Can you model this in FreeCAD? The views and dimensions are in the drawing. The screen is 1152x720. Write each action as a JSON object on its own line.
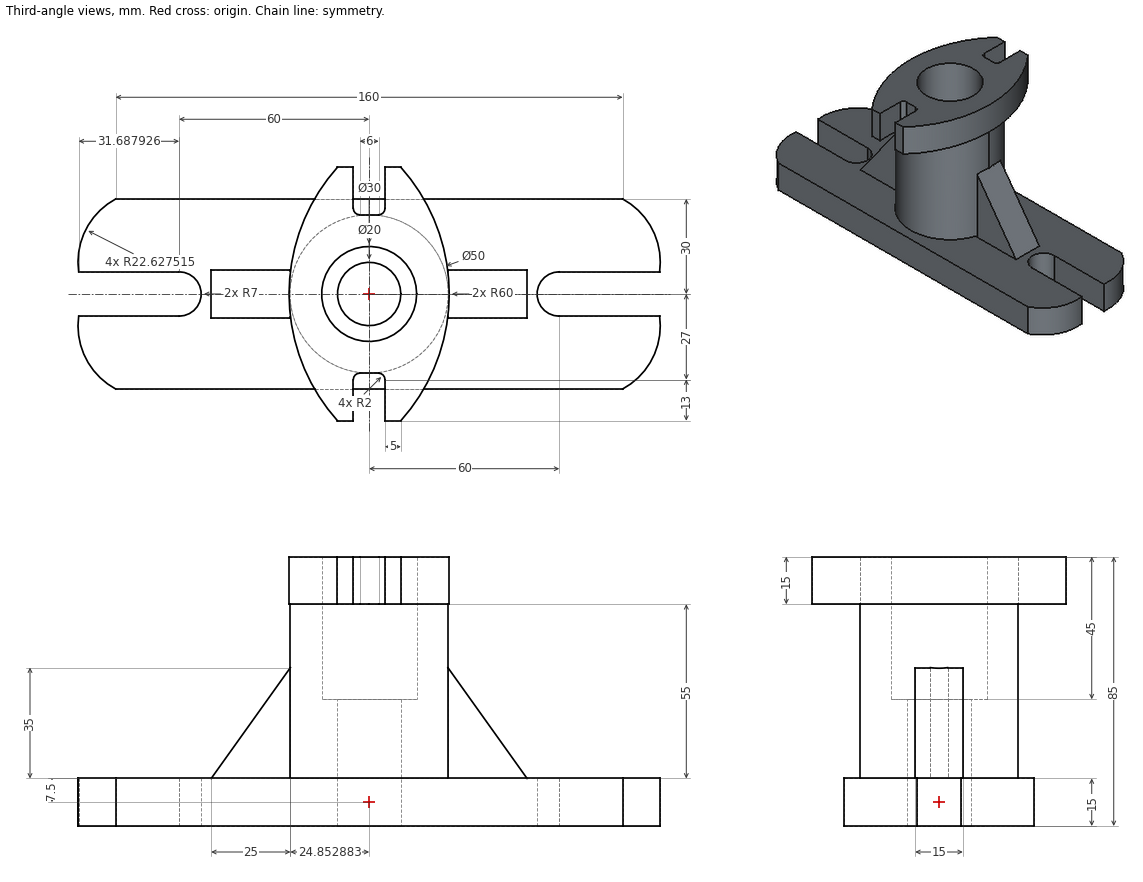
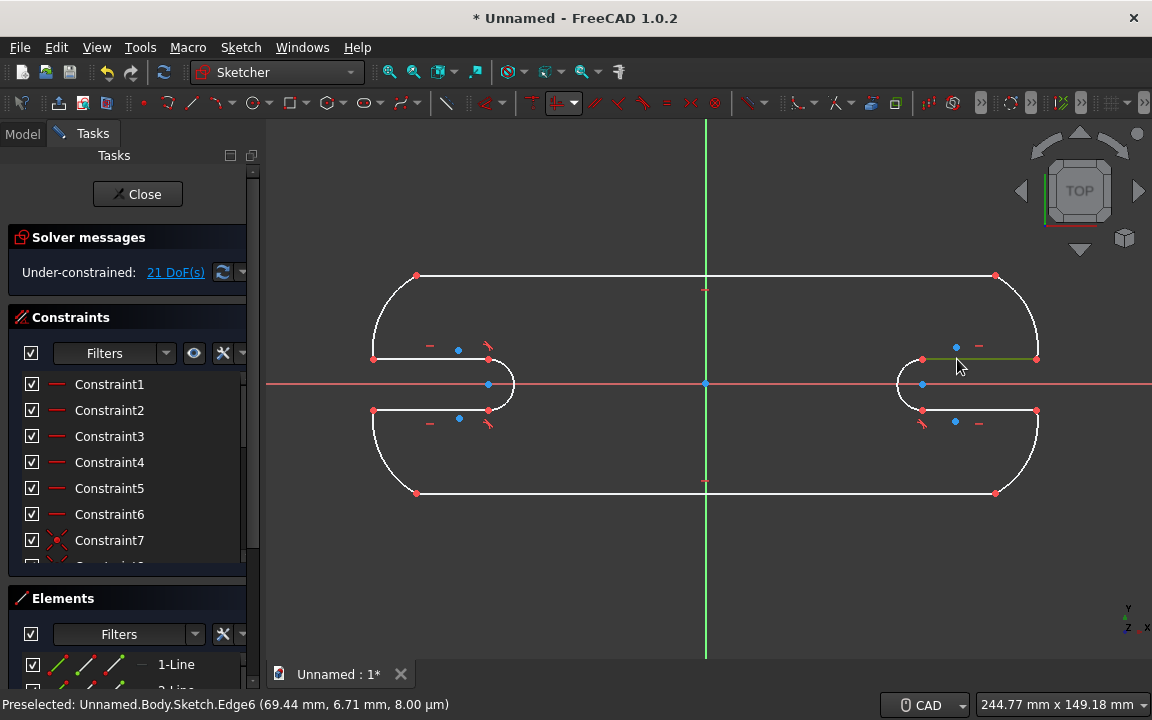
{"action": "left_click", "coordinate": [902, 370]}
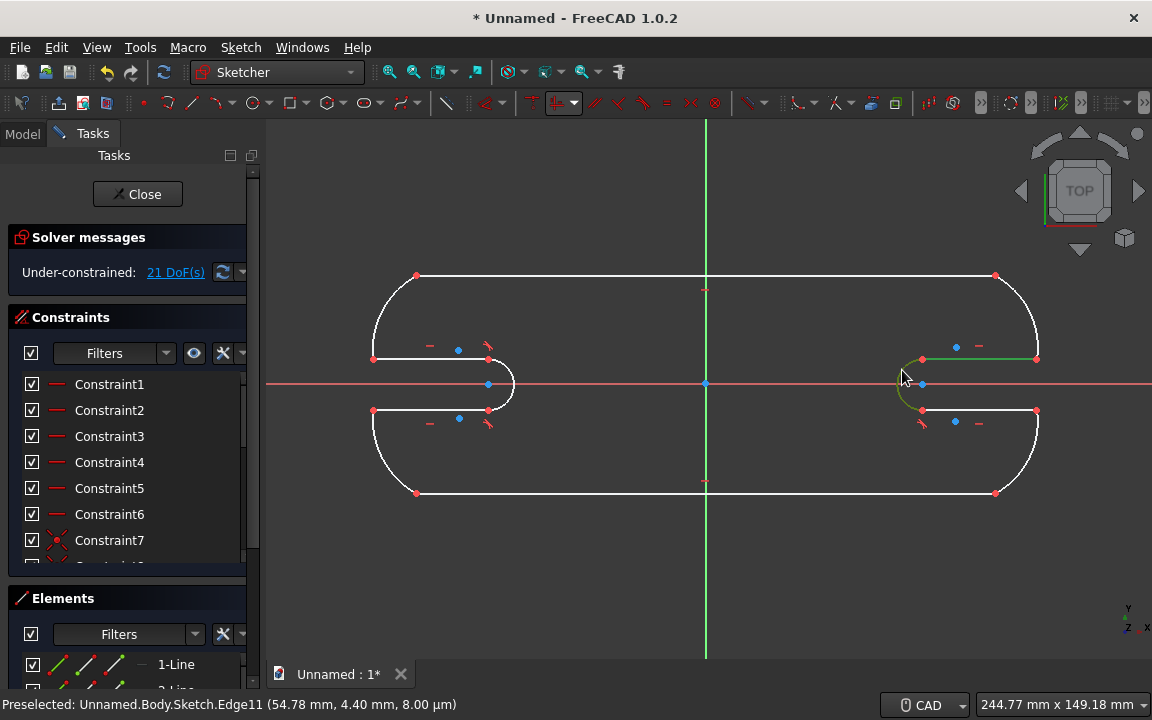
{"action": "key", "text": "t"}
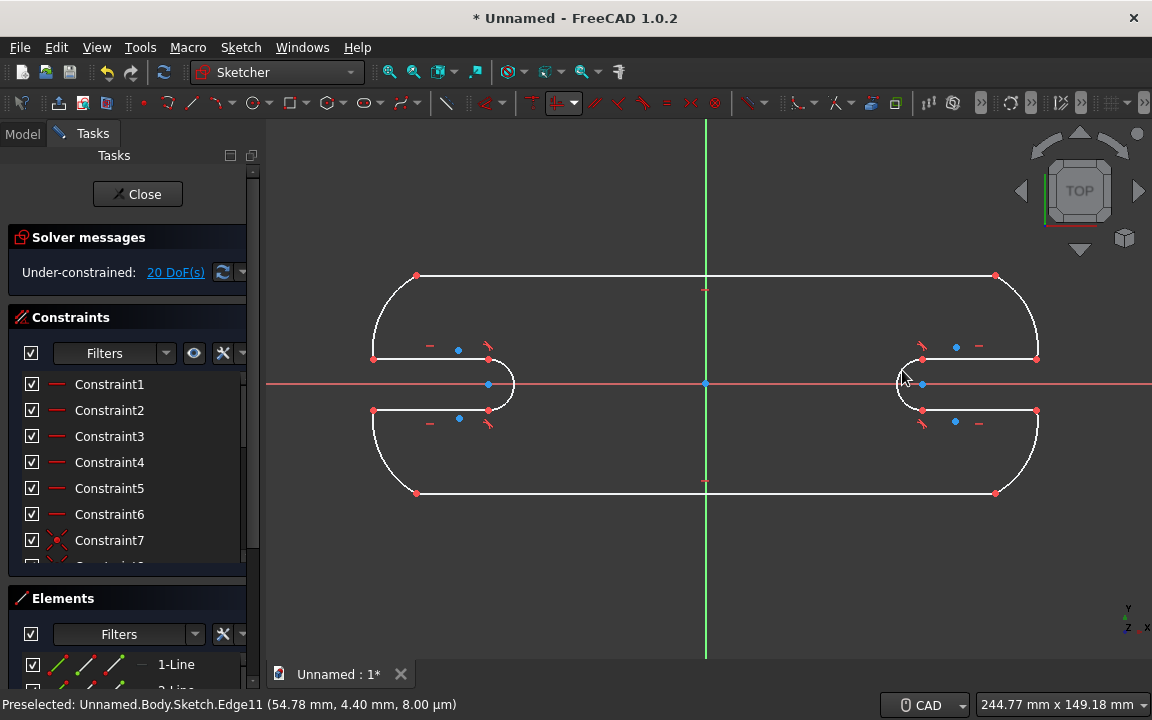
{"action": "left_click", "coordinate": [393, 295]}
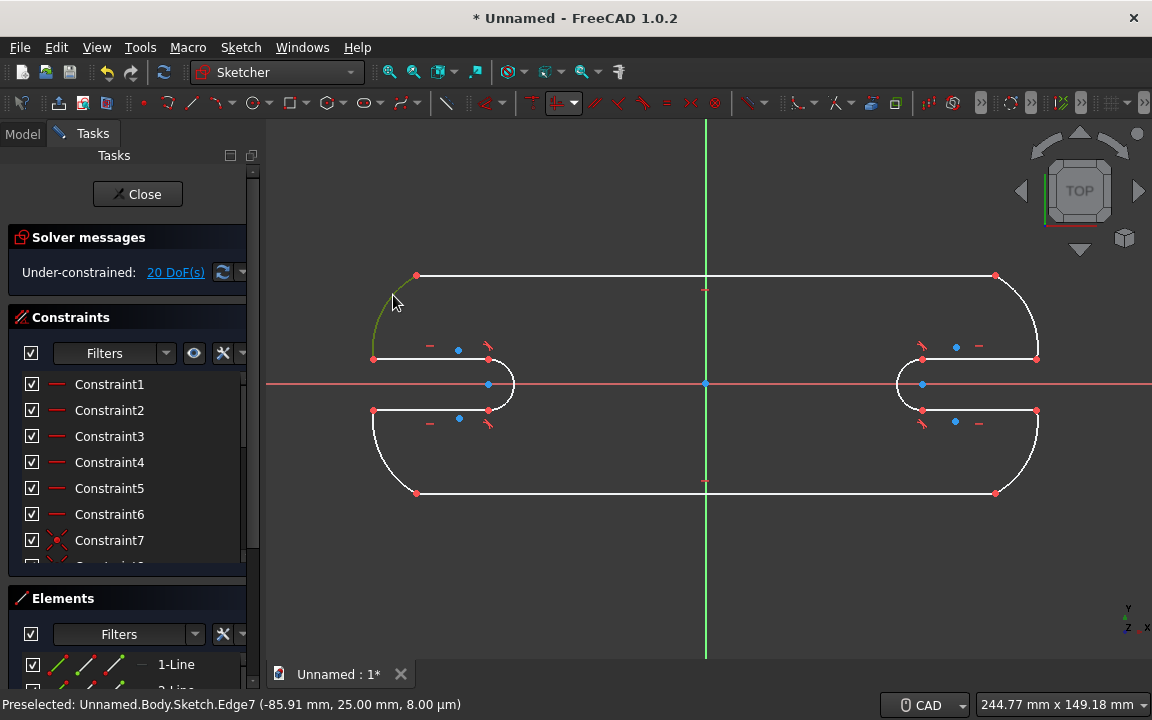
{"action": "left_click", "coordinate": [375, 440]}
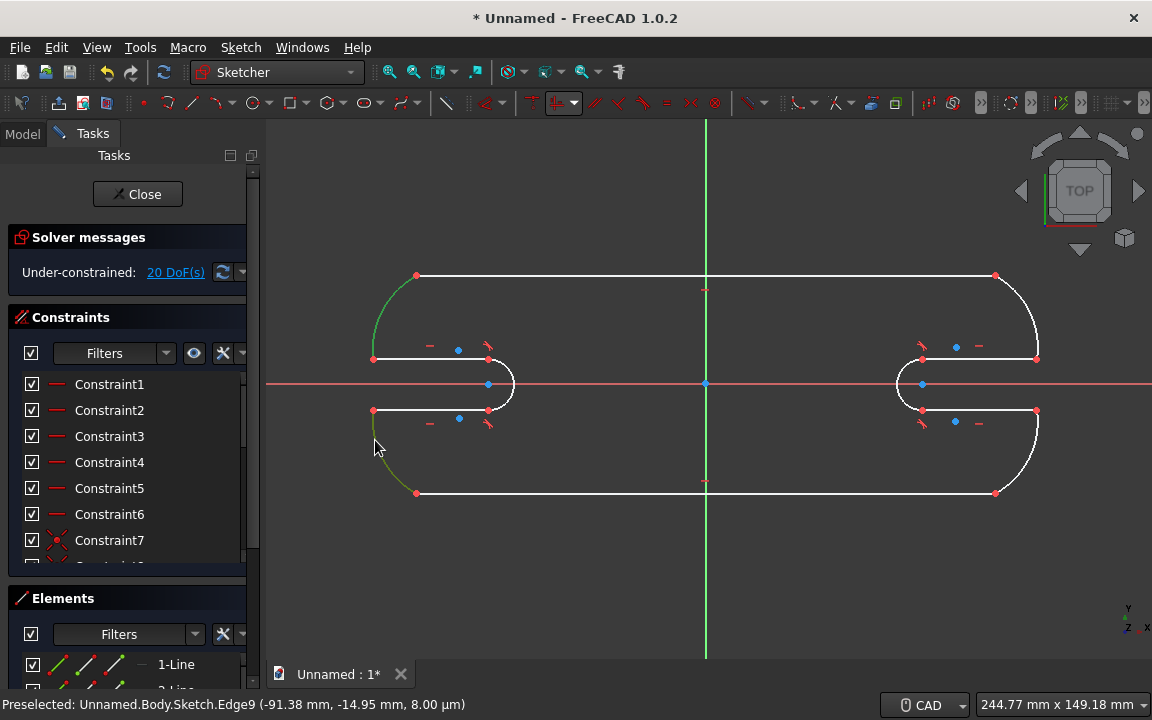
{"action": "scroll", "coordinate": [508, 400], "scroll_direction": "down", "scroll_amount": 2}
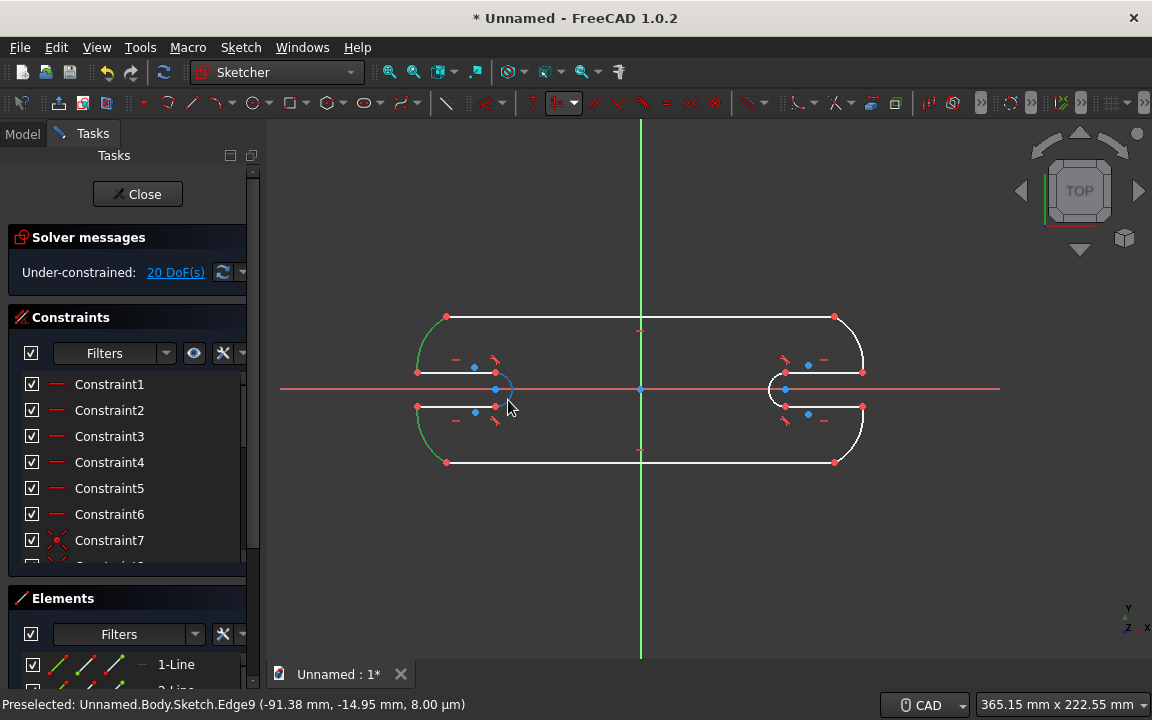
{"action": "left_click", "coordinate": [850, 450]}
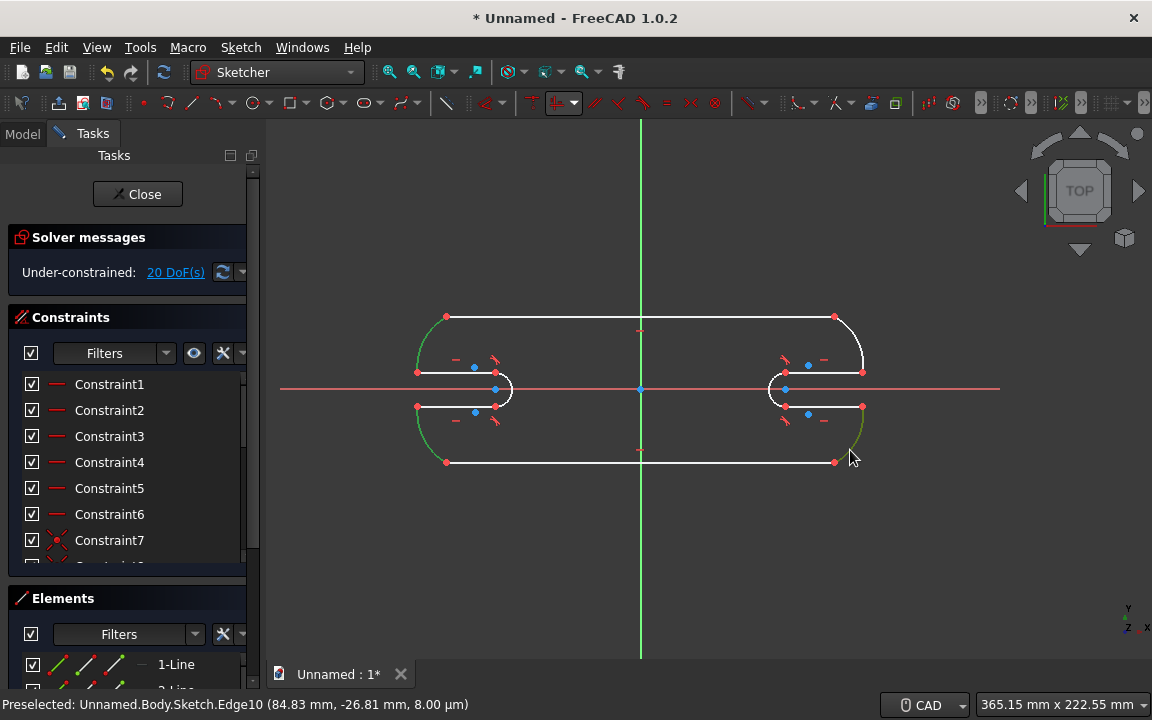
{"action": "left_click", "coordinate": [862, 353]}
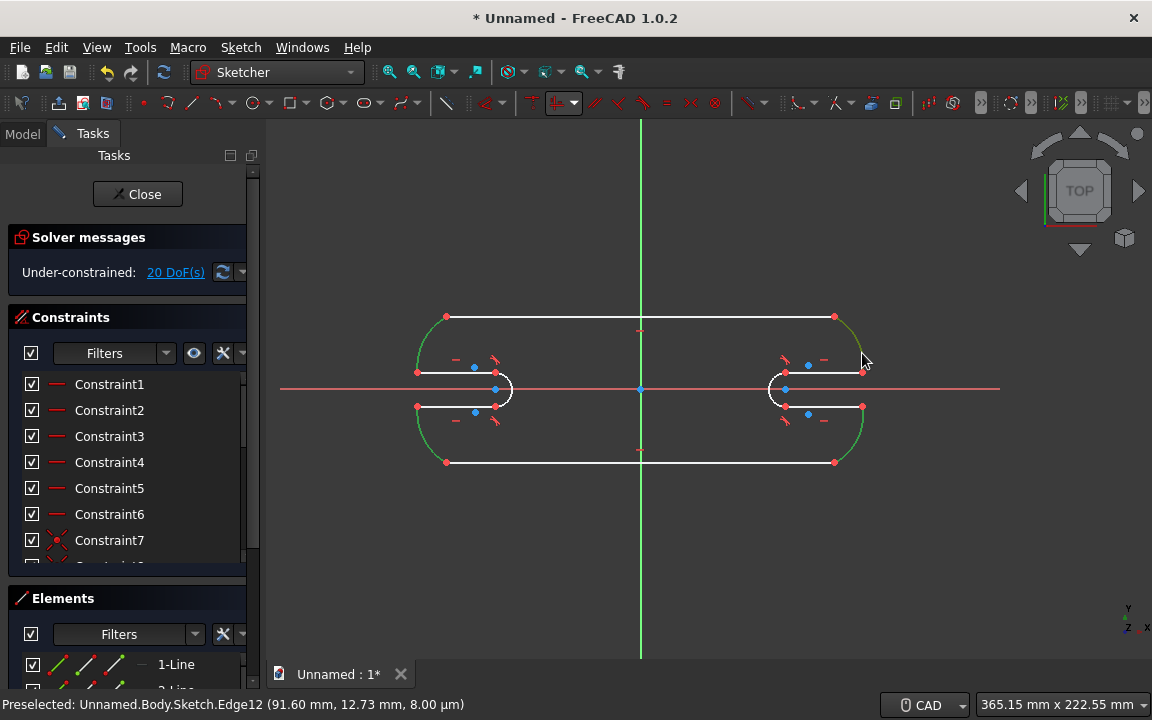
{"action": "key", "text": "e"}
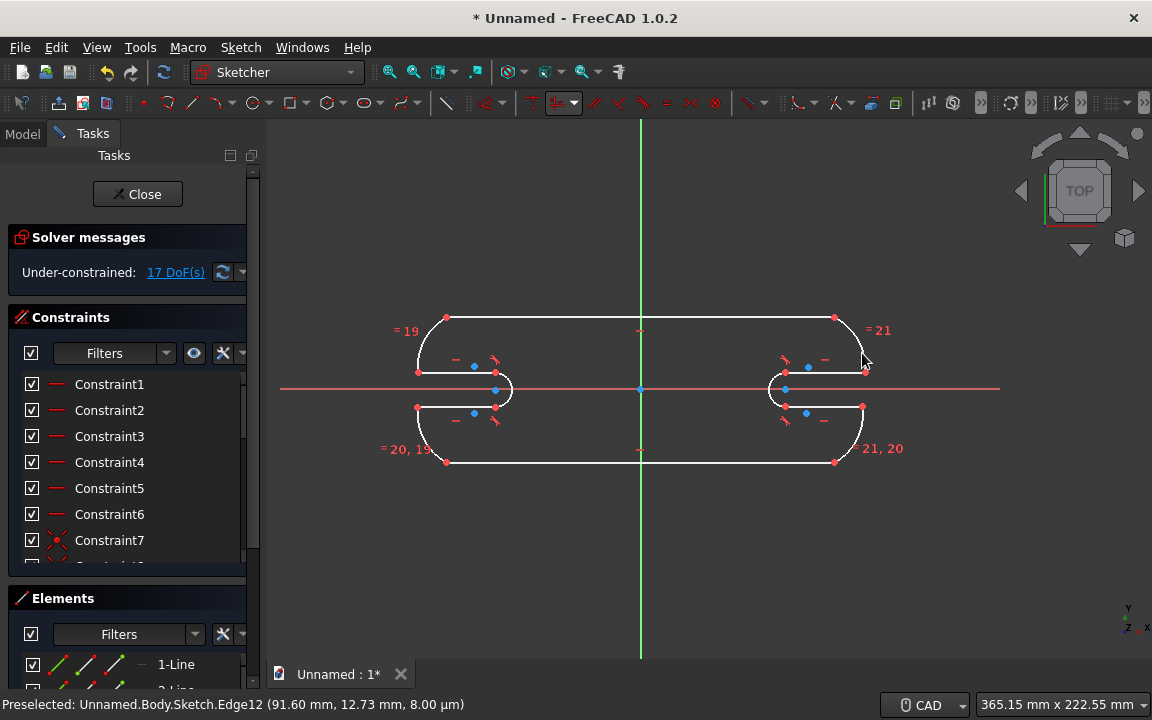
{"action": "scroll", "coordinate": [509, 400], "scroll_direction": "up", "scroll_amount": 2}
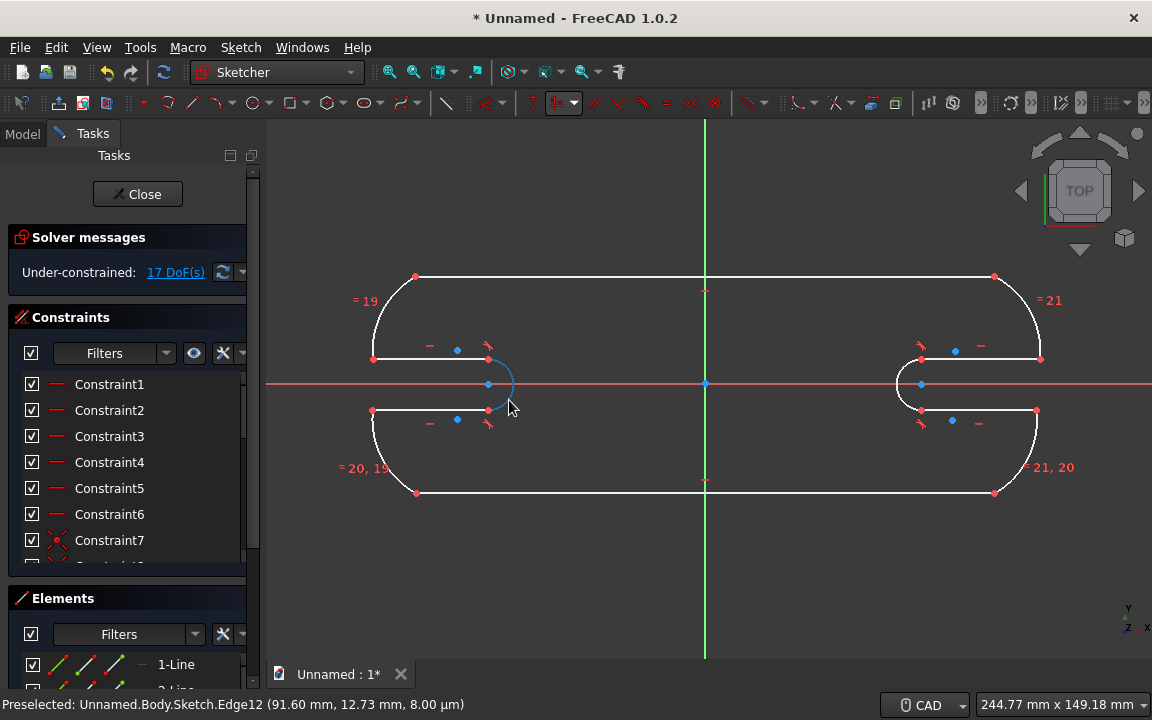
{"action": "left_click", "coordinate": [509, 400]}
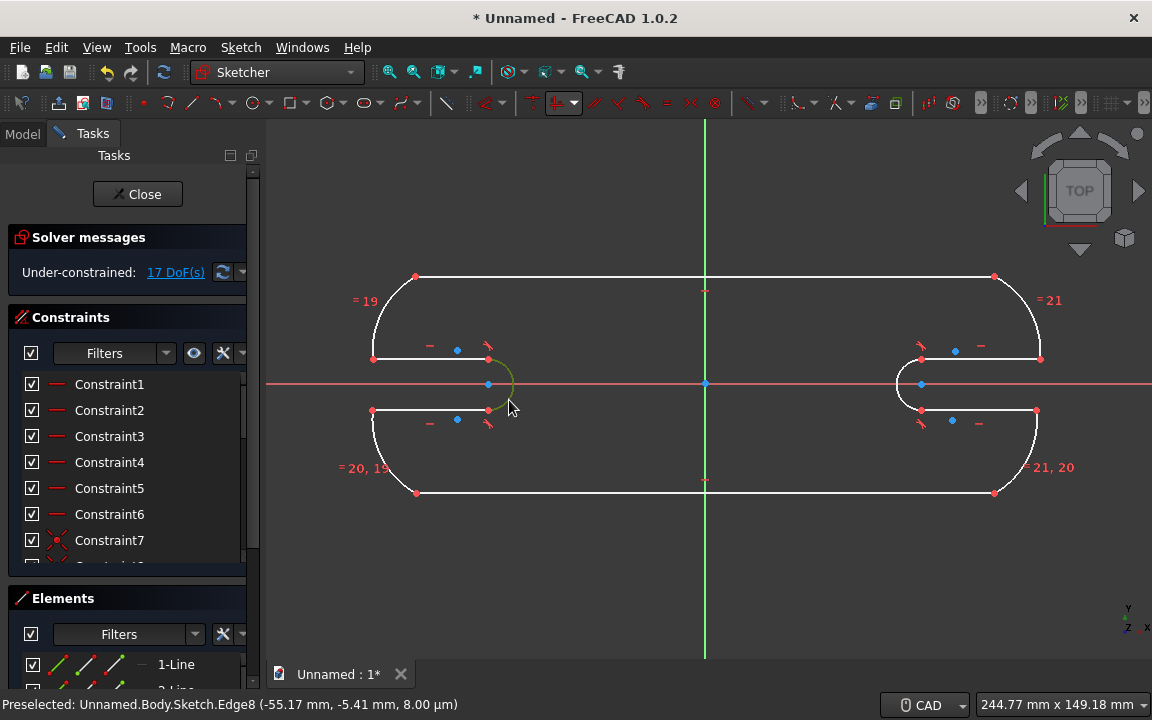
{"action": "left_click", "coordinate": [901, 370]}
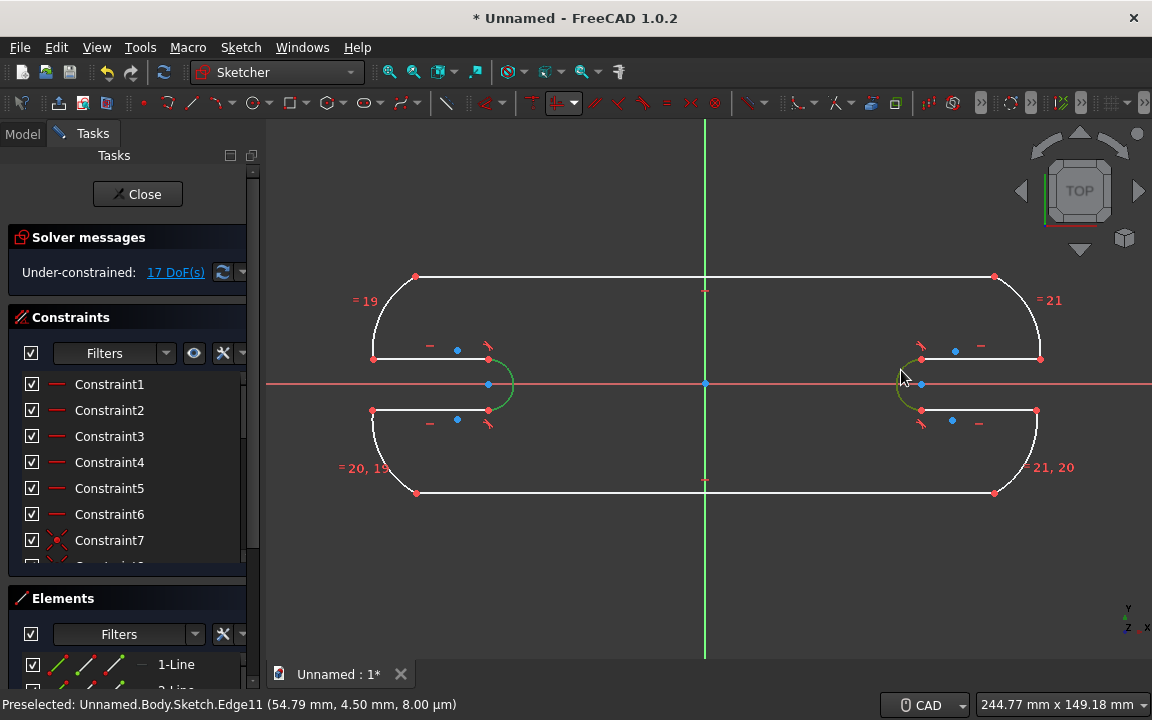
{"action": "key", "text": "e"}